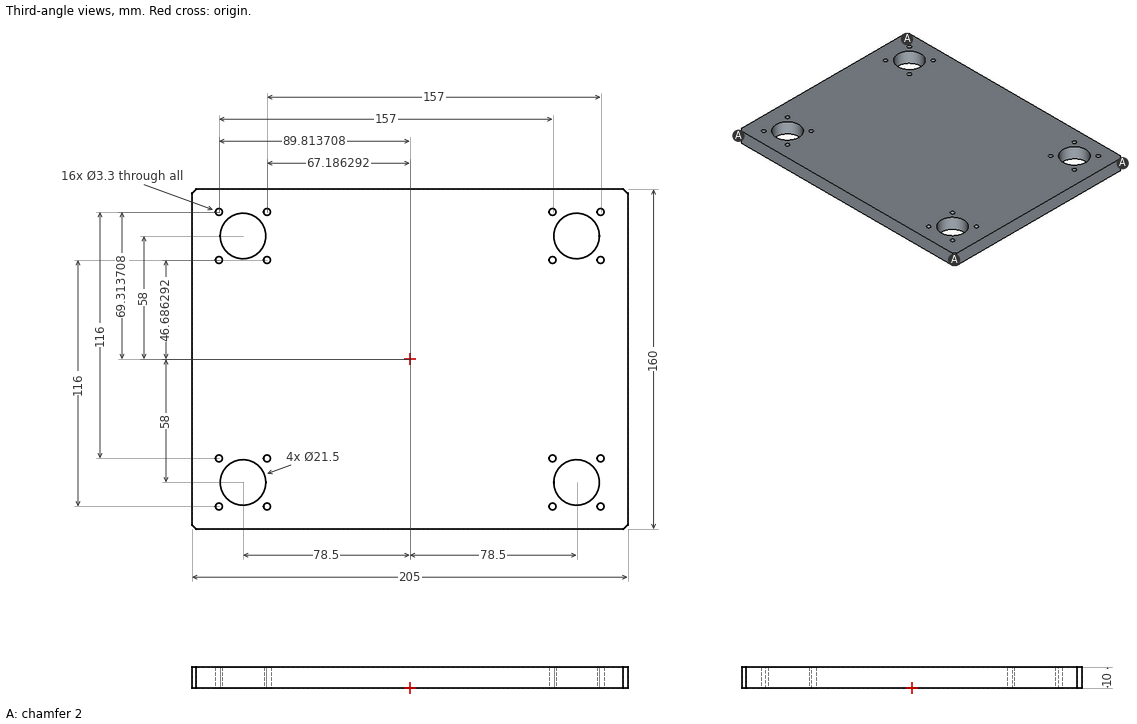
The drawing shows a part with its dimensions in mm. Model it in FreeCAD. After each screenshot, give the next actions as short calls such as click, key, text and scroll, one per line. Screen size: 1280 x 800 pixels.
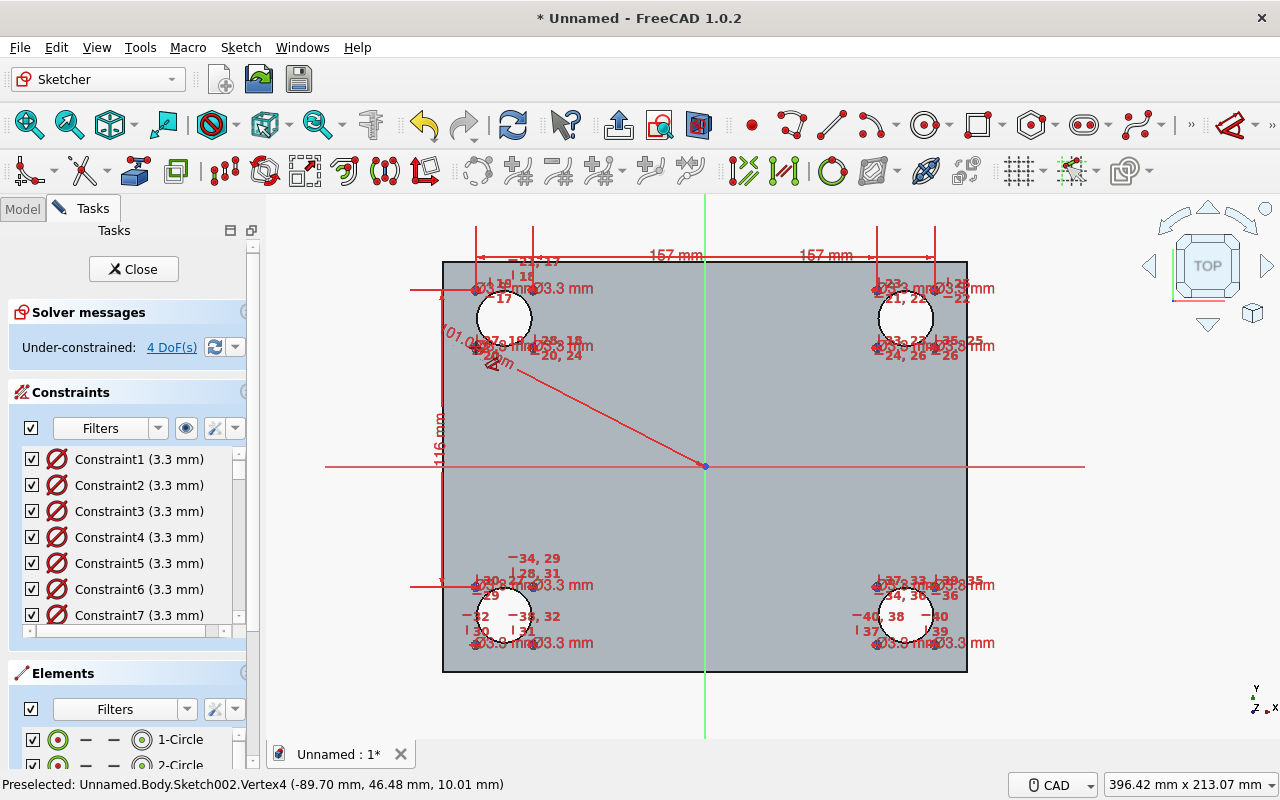
click(476, 645)
click(442, 496)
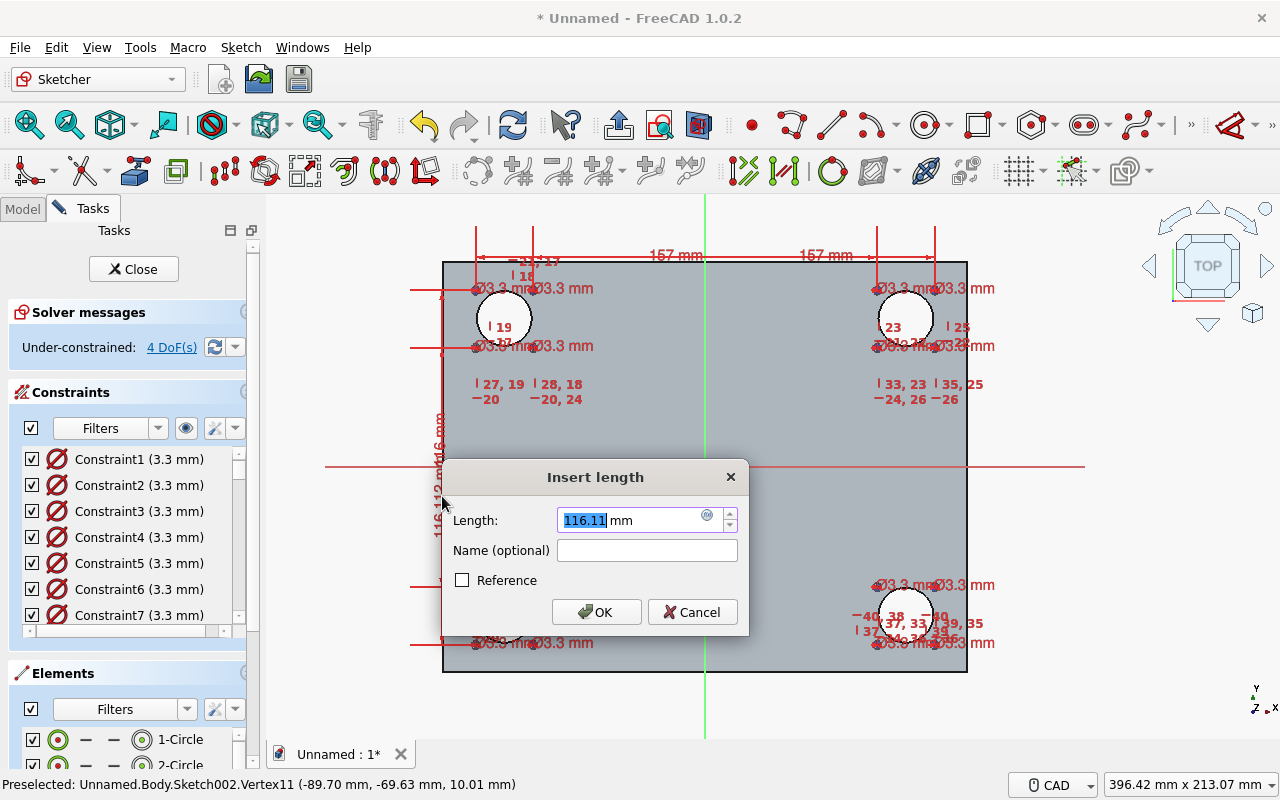
text(116)
key(Return)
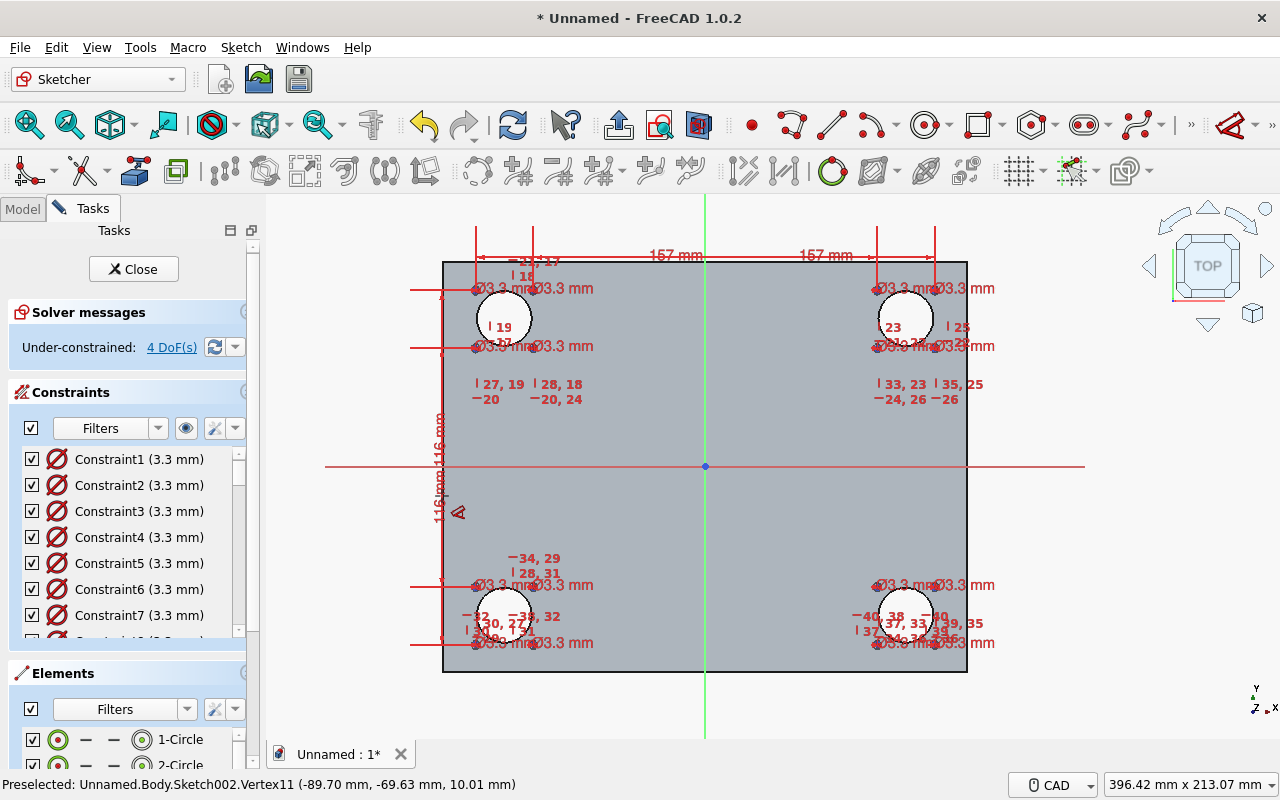
click(476, 290)
click(590, 256)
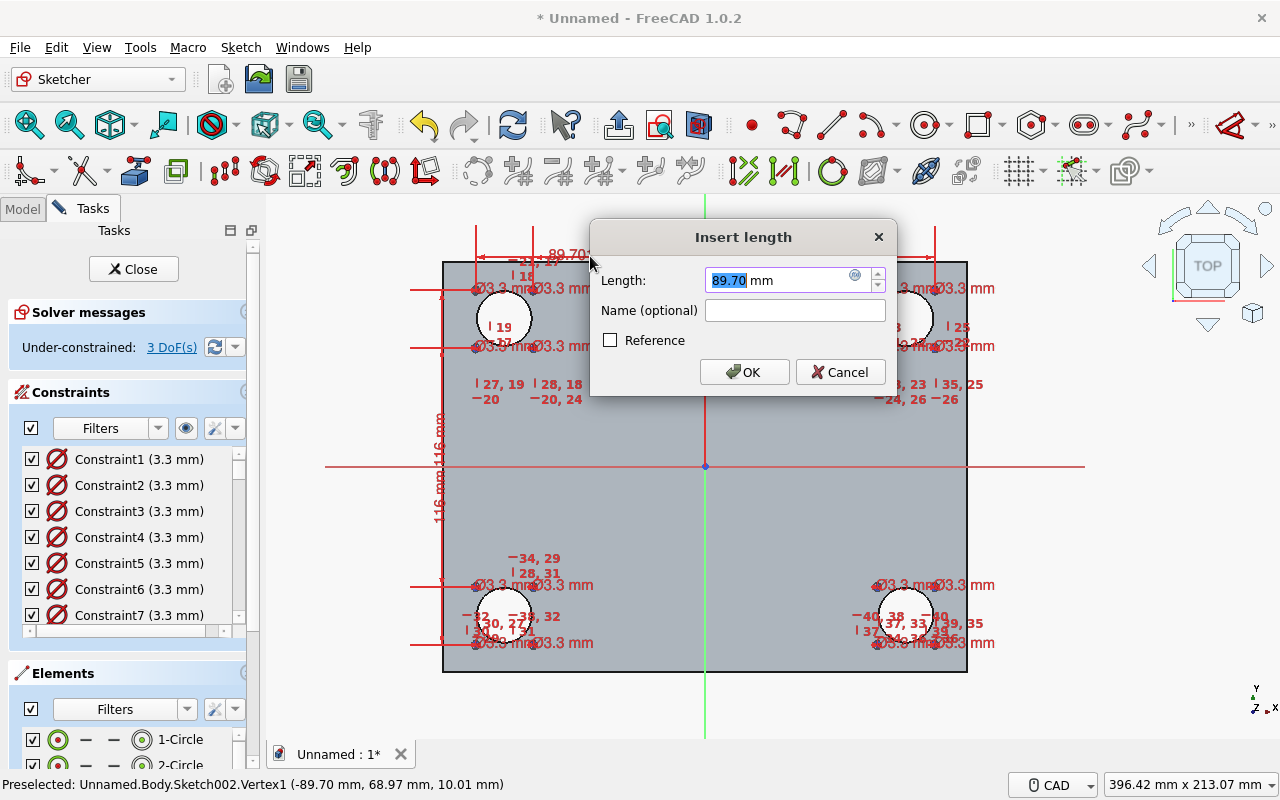
text(89.813708)
key(Return)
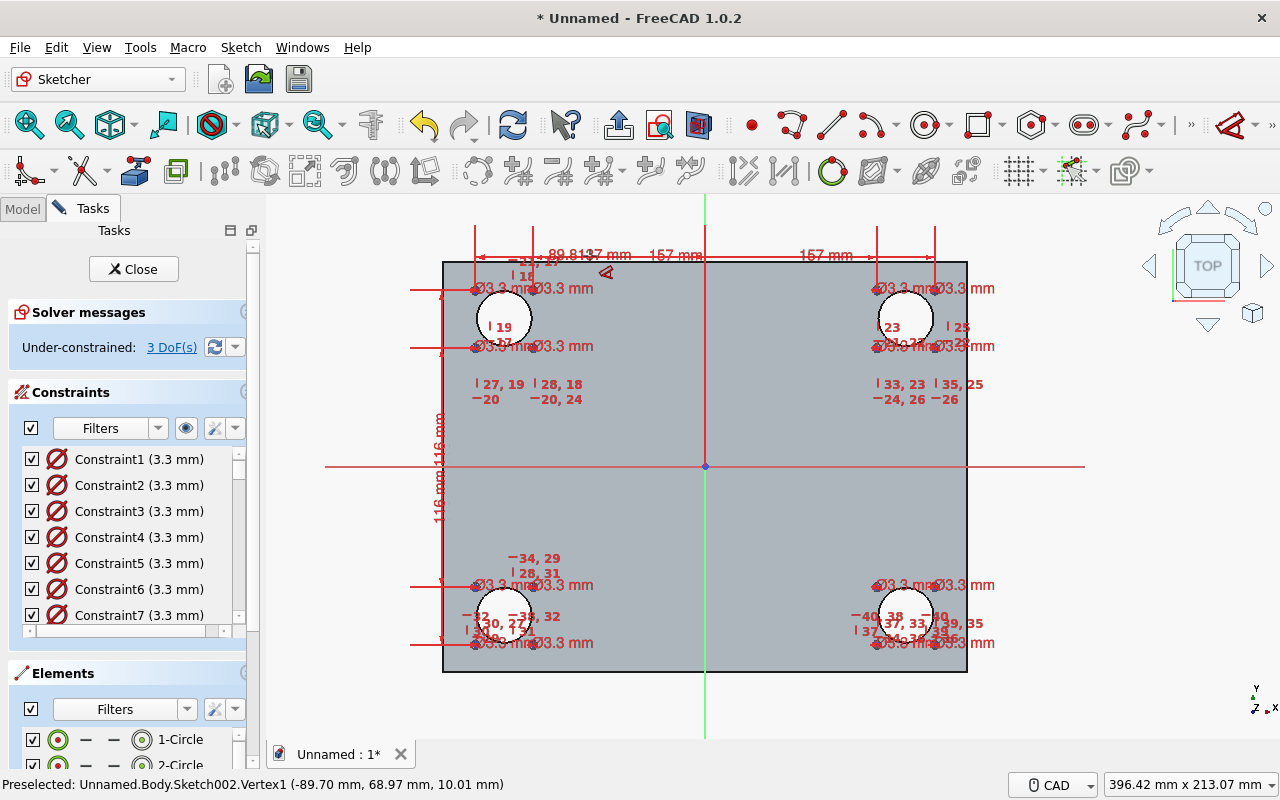
click(475, 290)
click(441, 379)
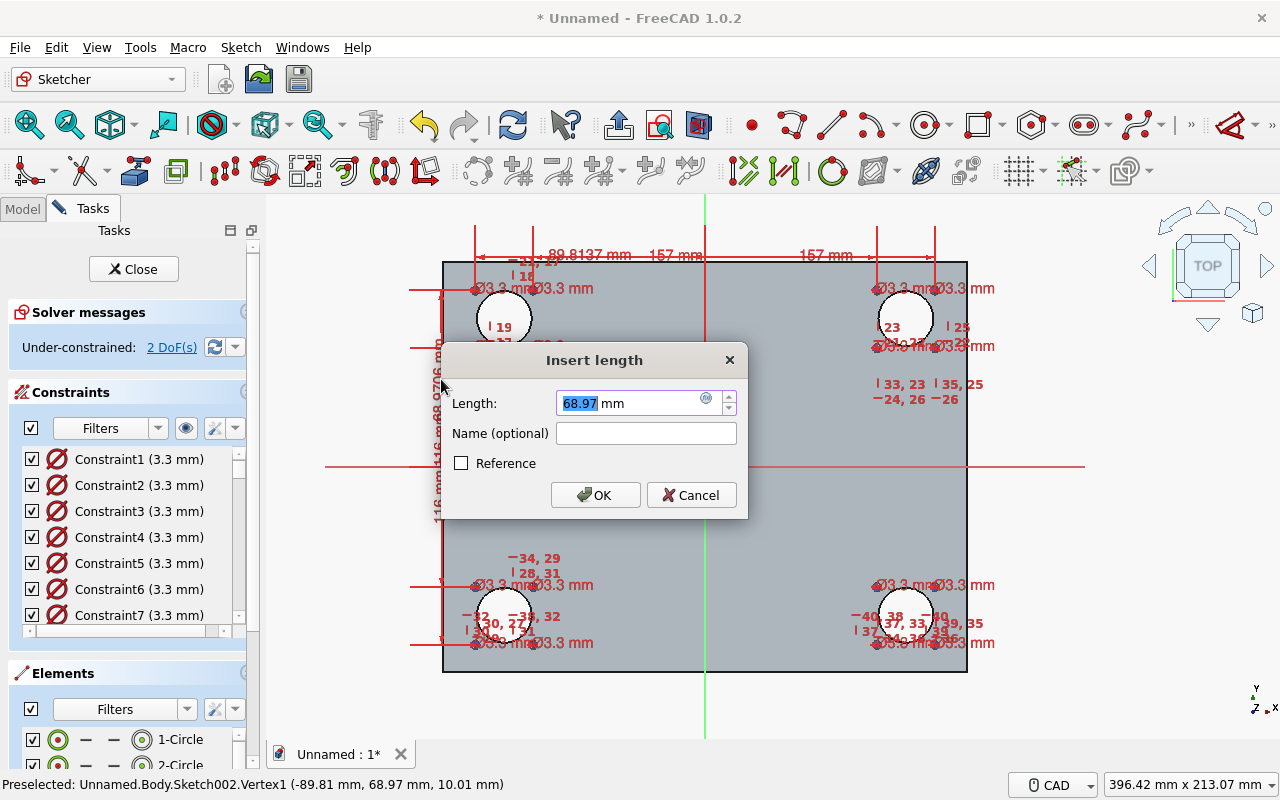
text(69.313708)
key(Return)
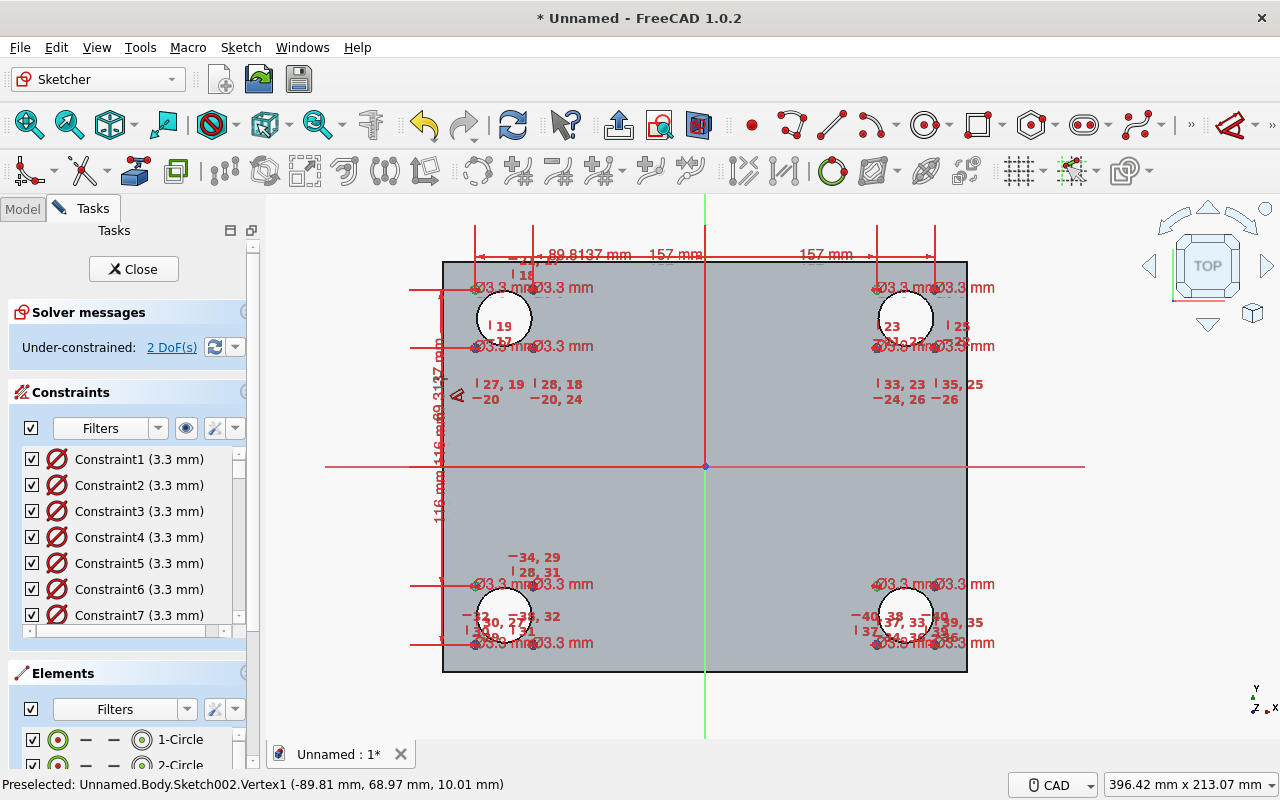
click(533, 290)
click(619, 501)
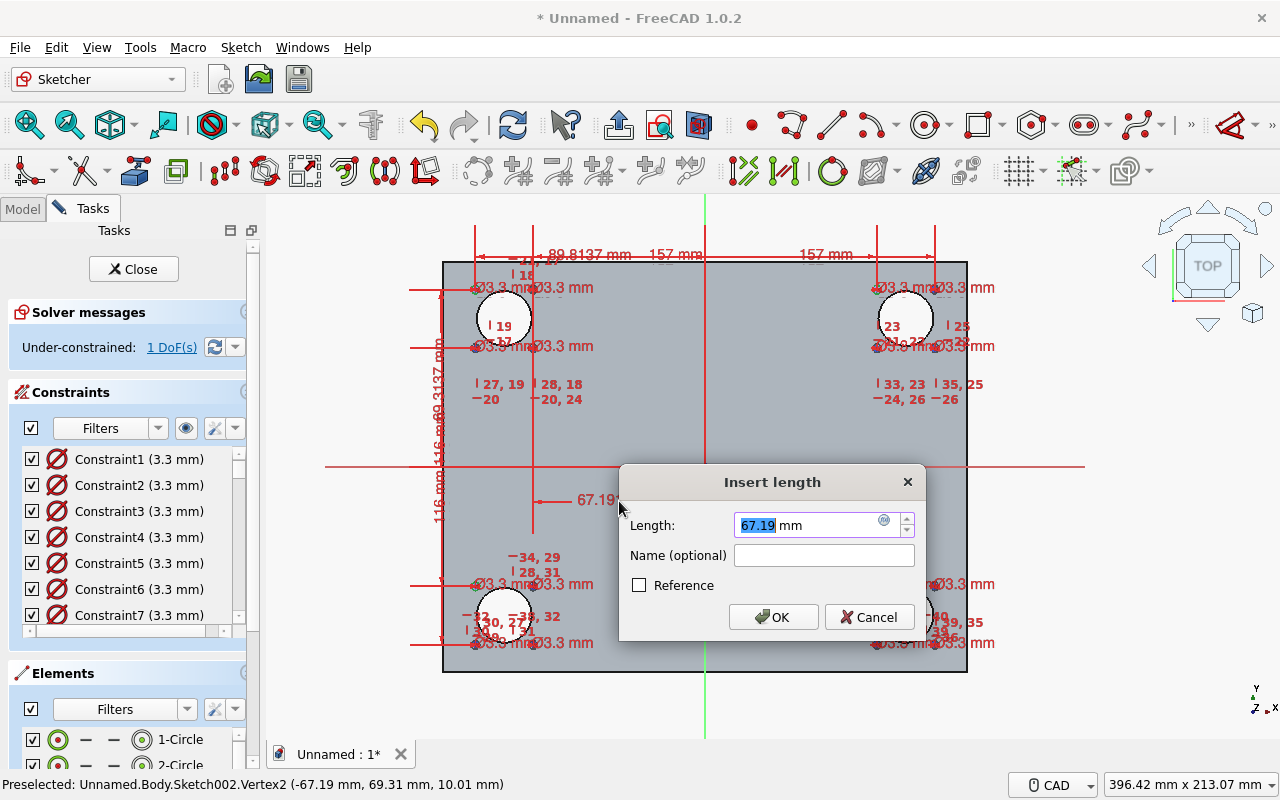
text(67.186292)
key(Return)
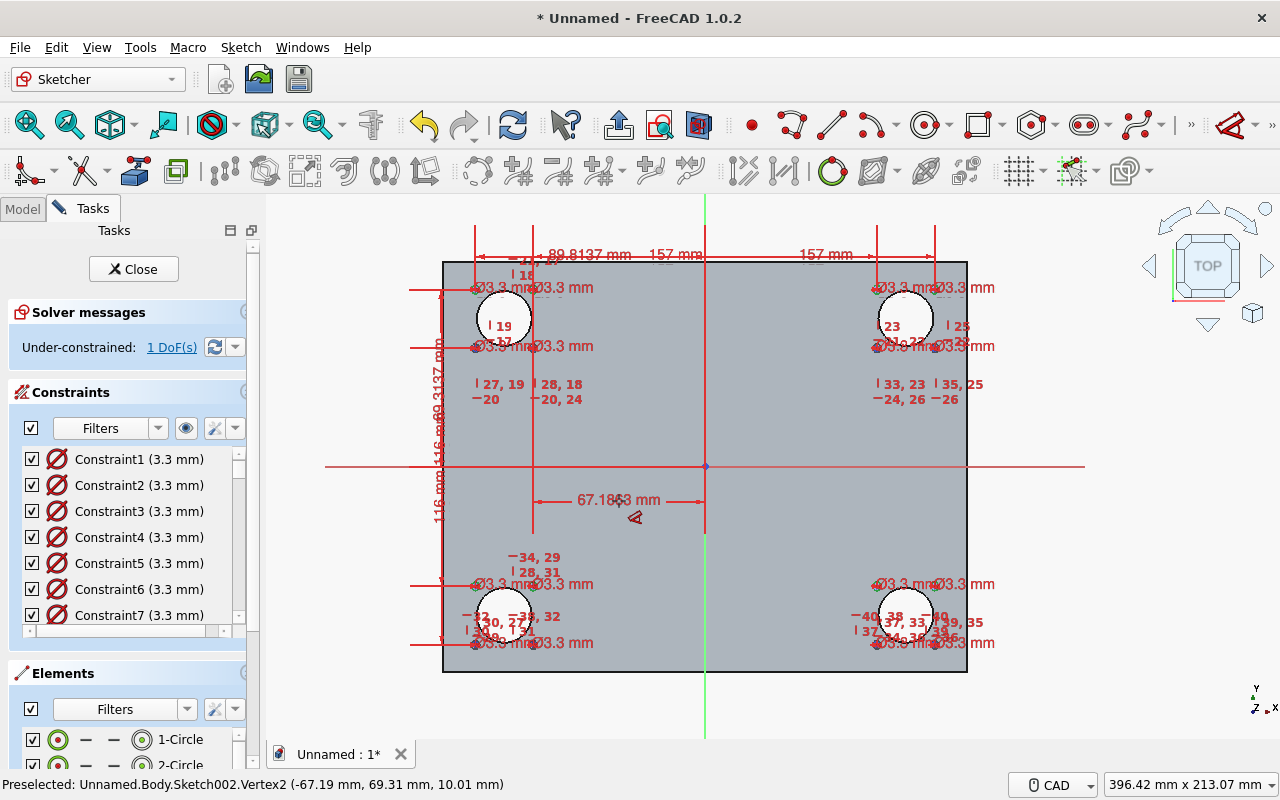
click(533, 348)
click(499, 408)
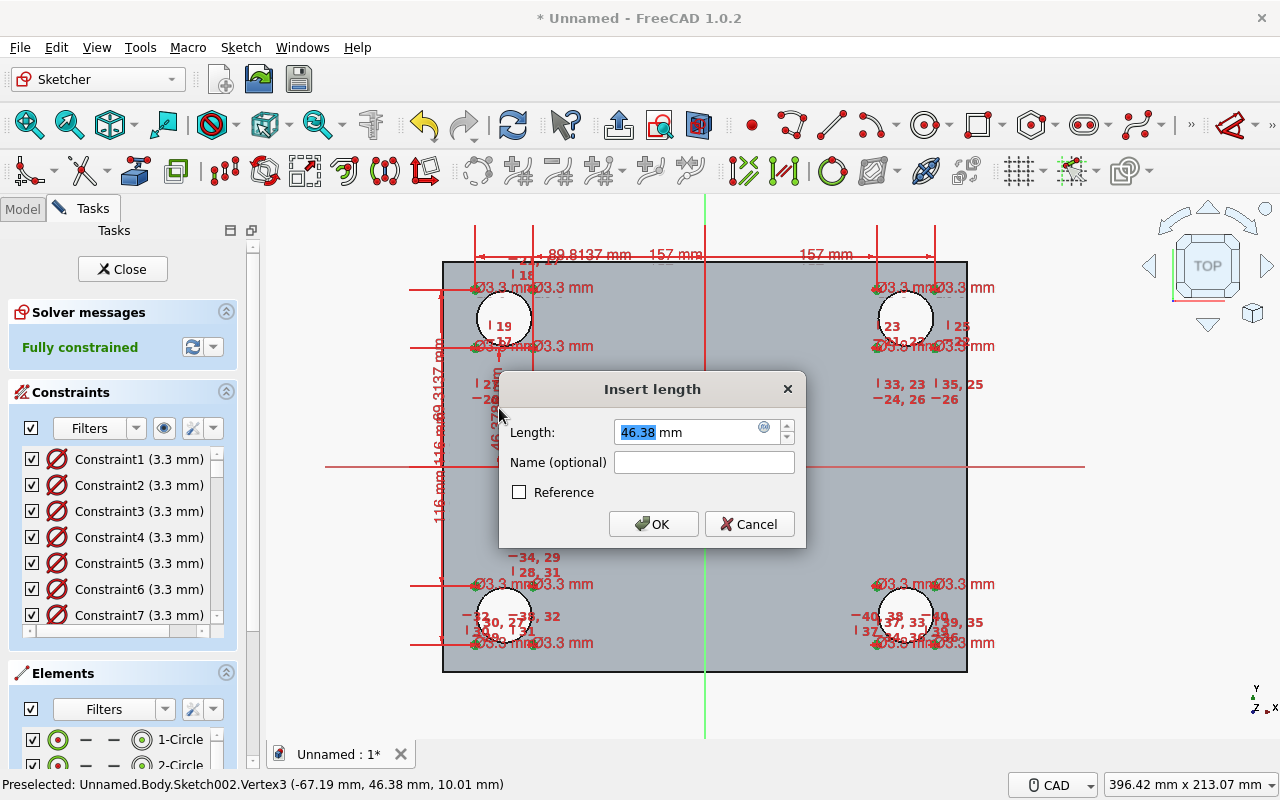
text(46.686292)
key(Return)
key(Escape)